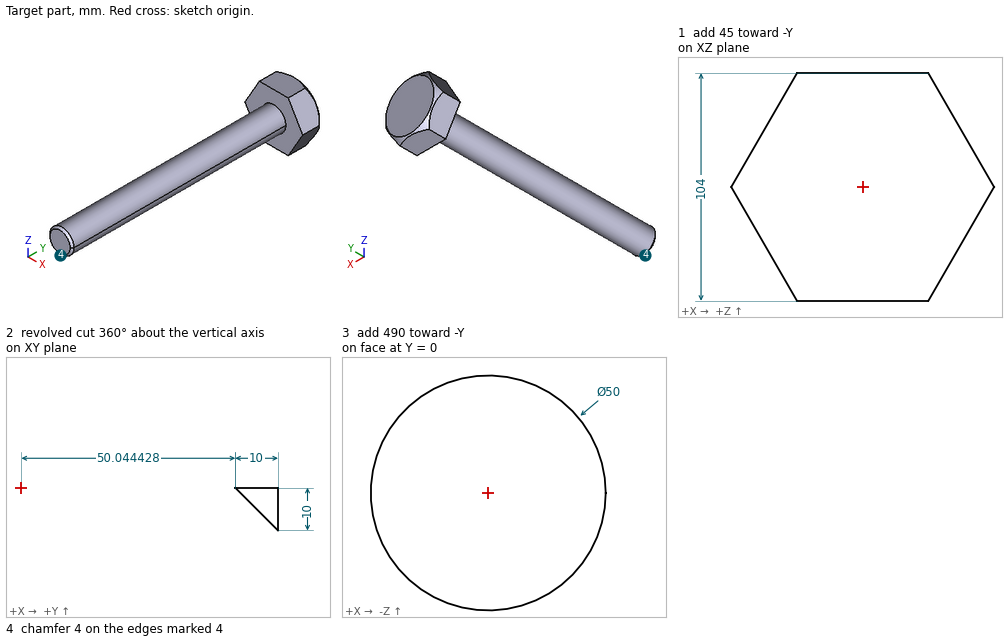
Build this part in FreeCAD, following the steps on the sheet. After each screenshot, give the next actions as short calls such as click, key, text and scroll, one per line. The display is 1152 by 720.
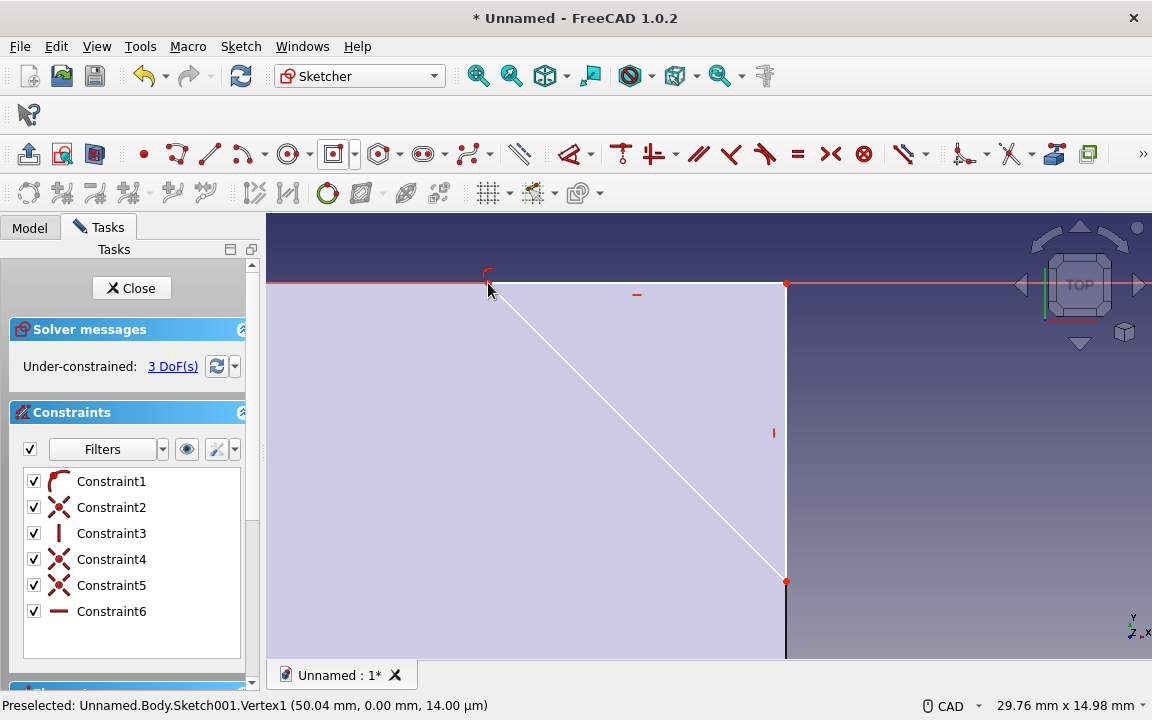
click(786, 492)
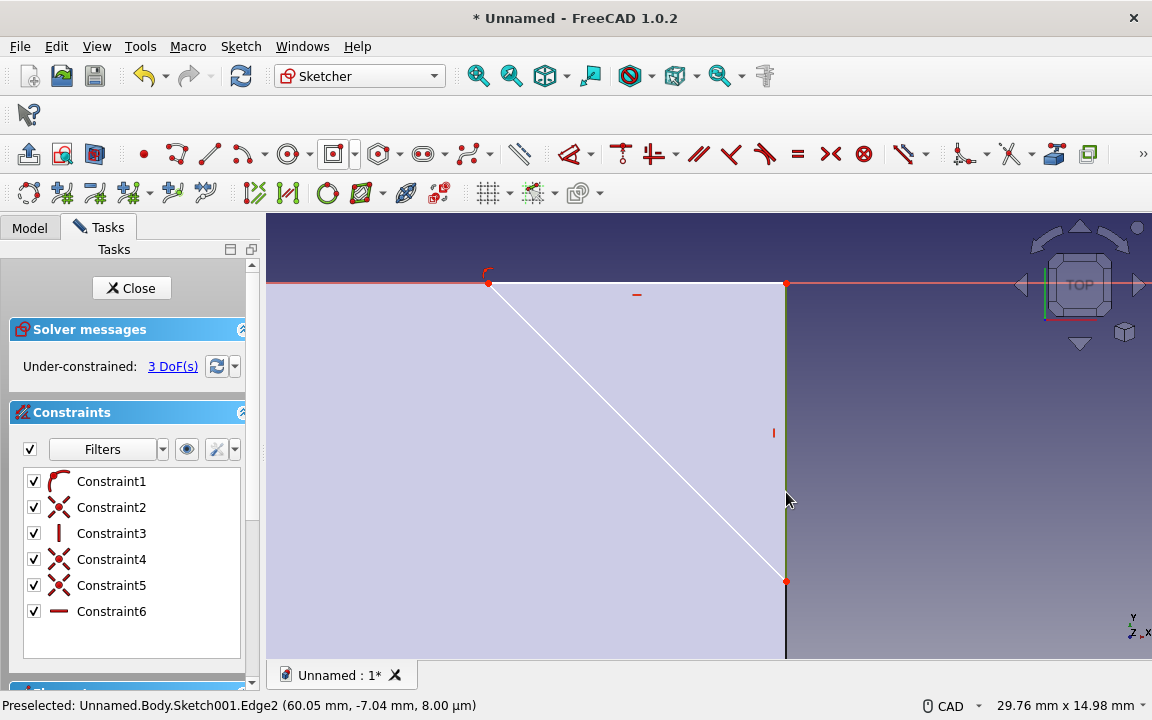
key(i)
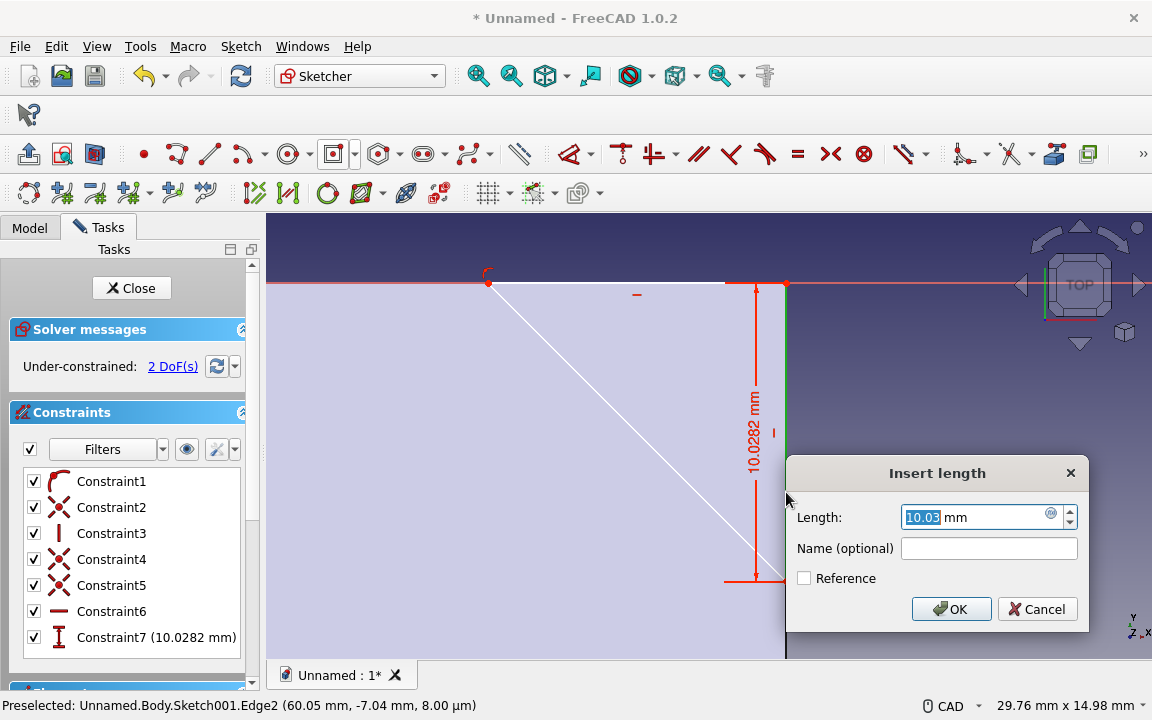
text(10)
key(Return)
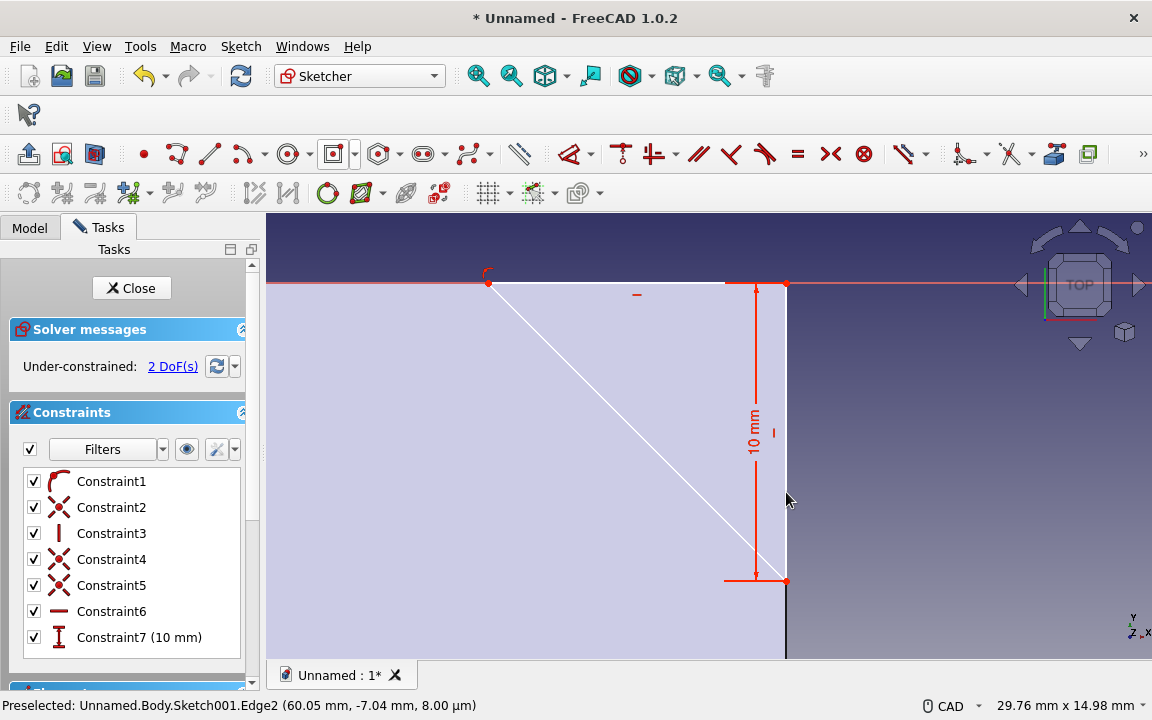
click(697, 283)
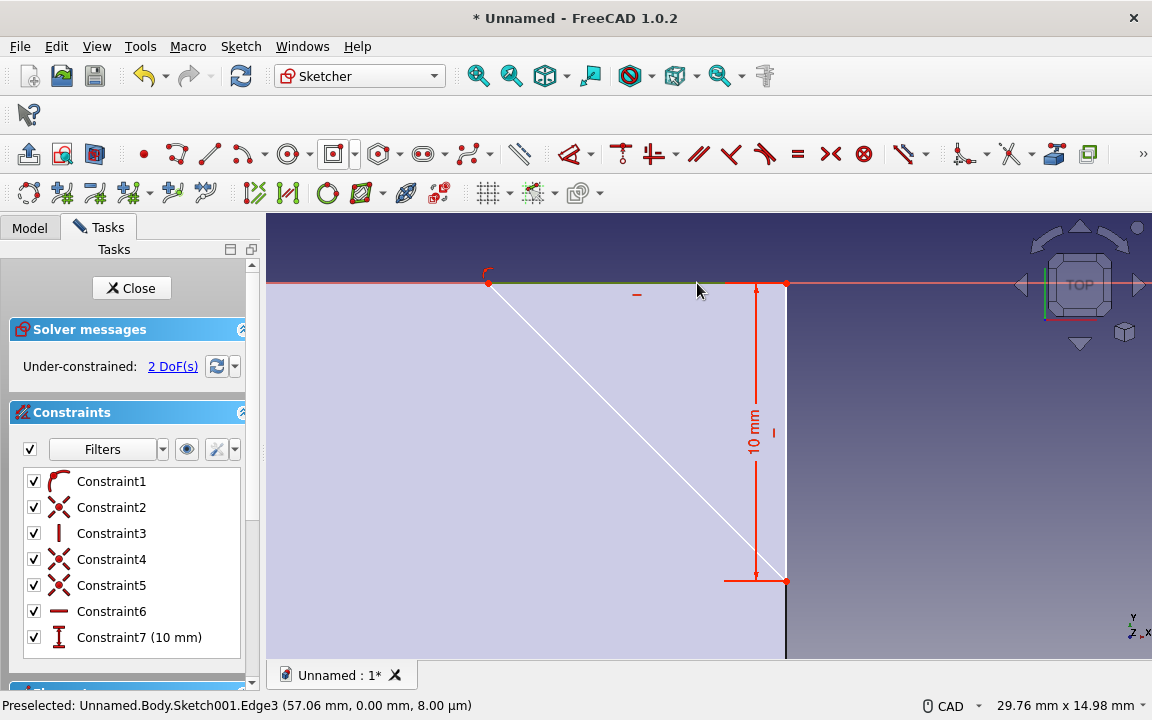
key(l)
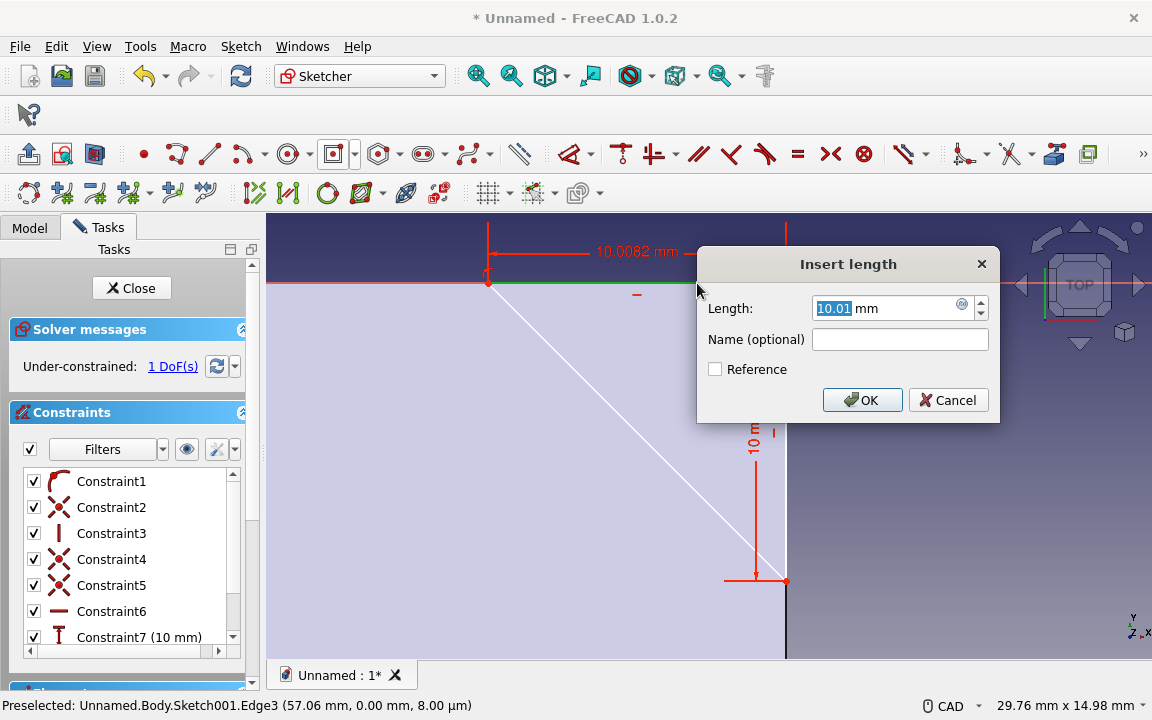
text(10)
key(Return)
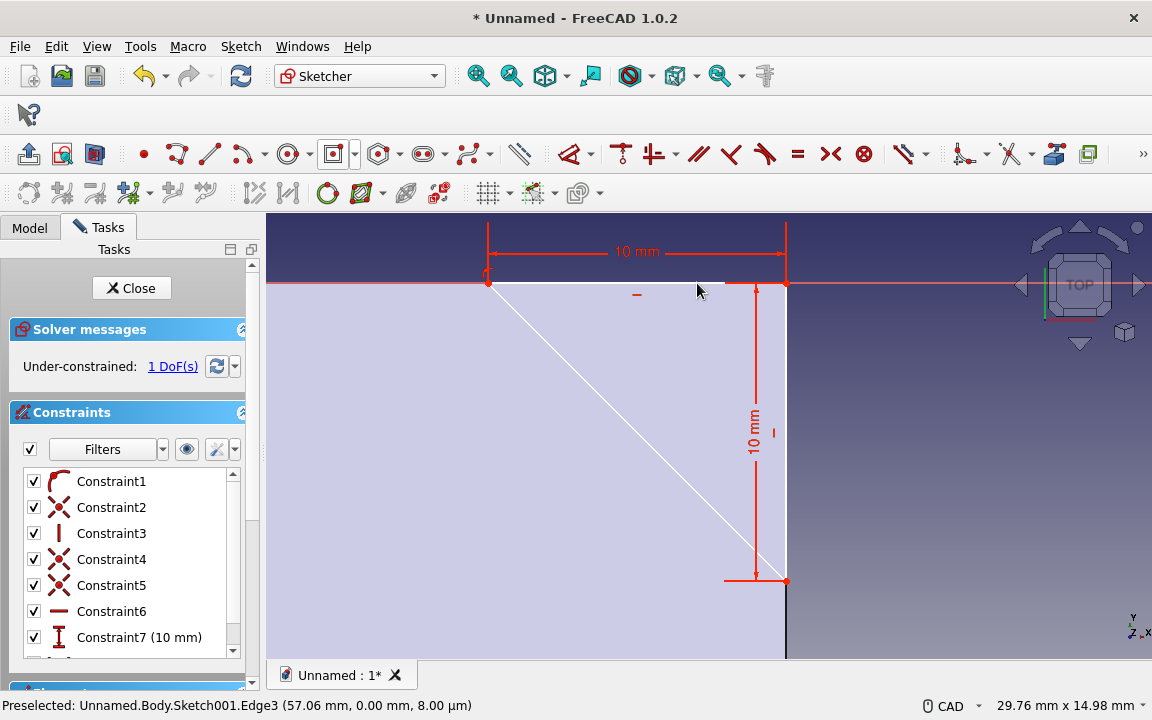
click(488, 283)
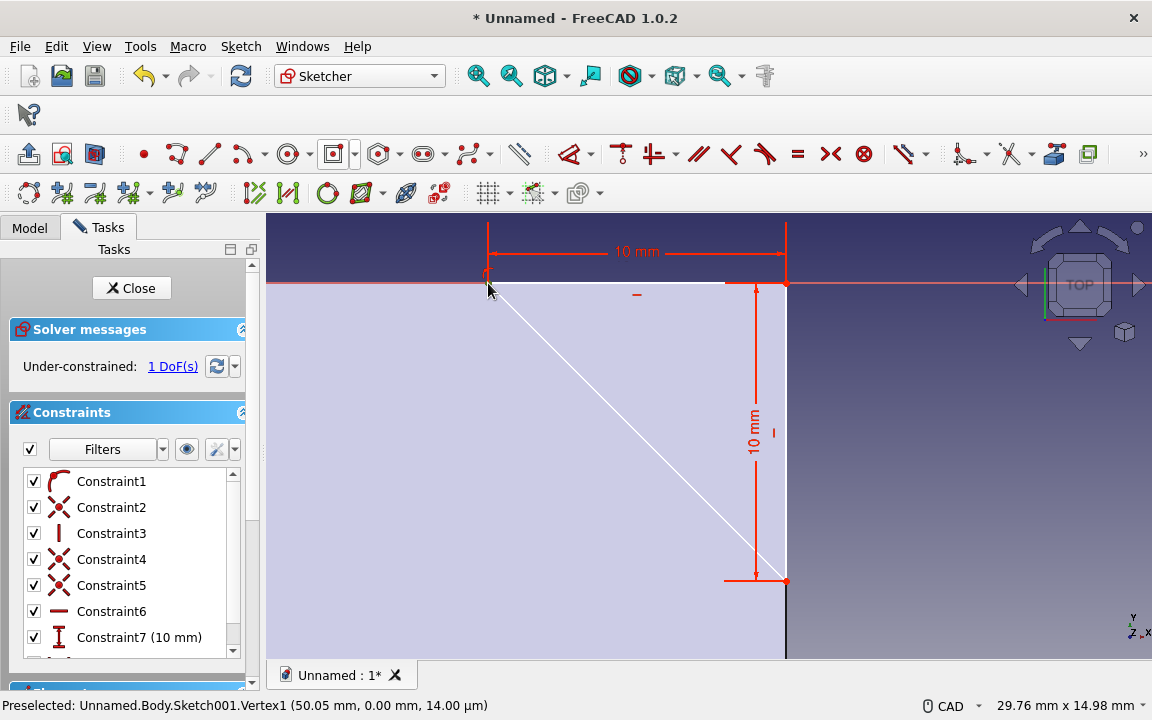
key(l)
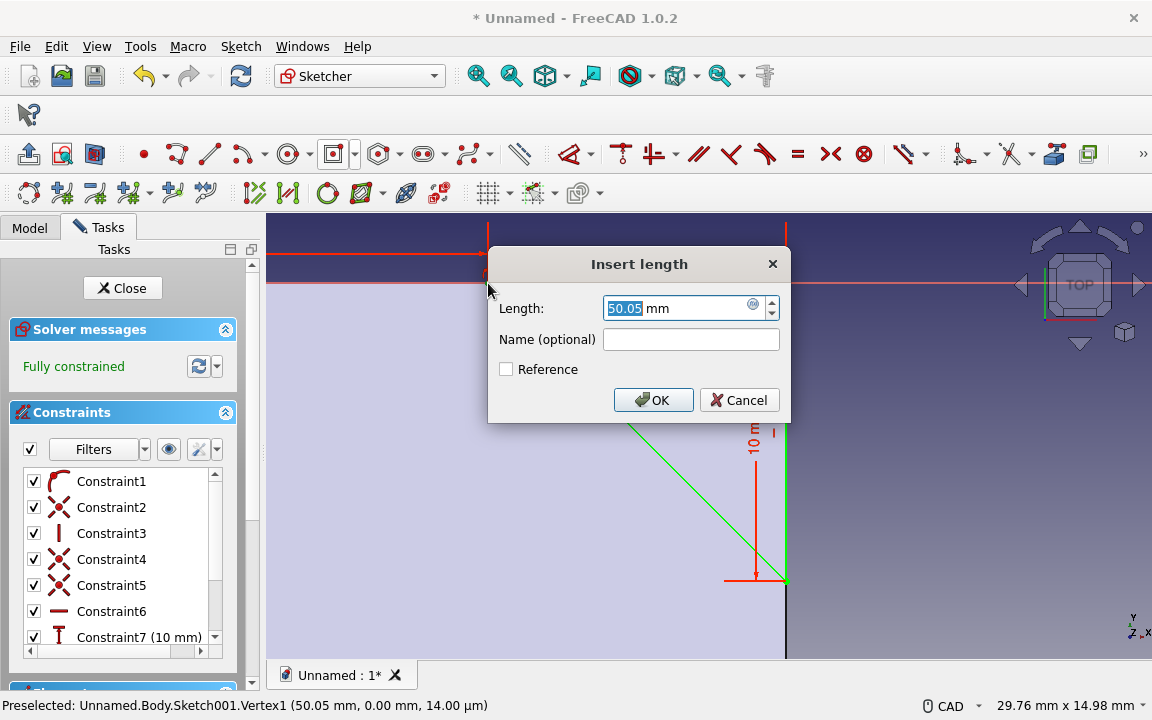
text(50.044428)
key(Return)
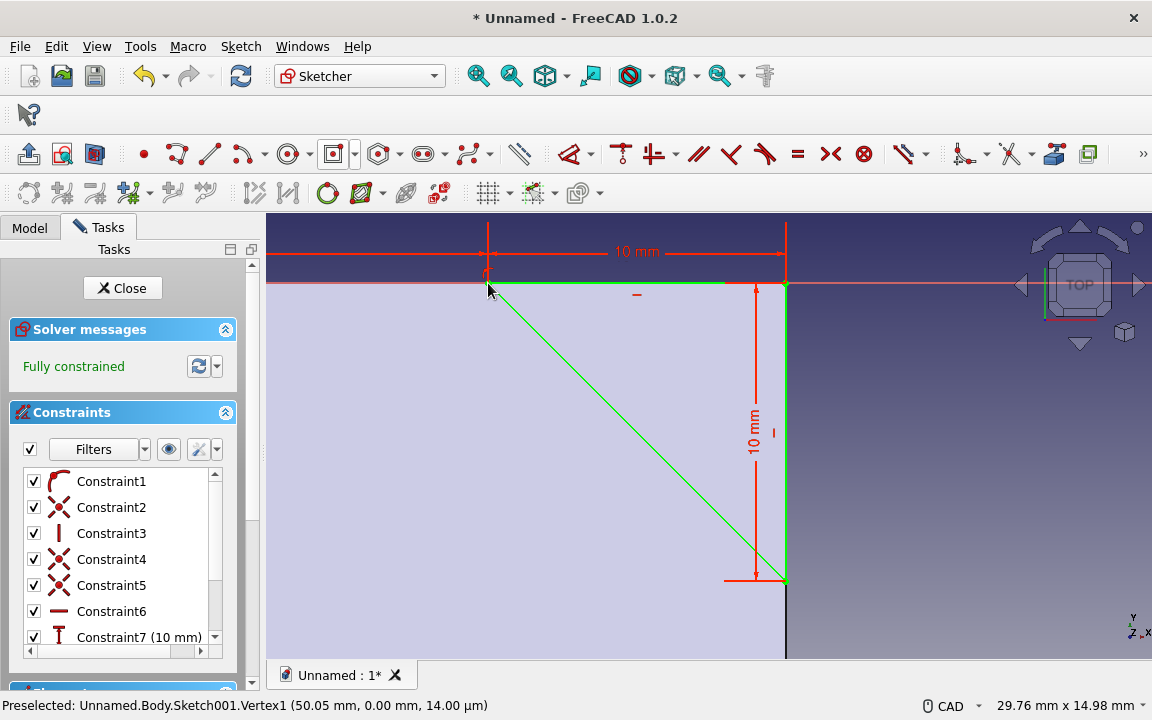
click(123, 288)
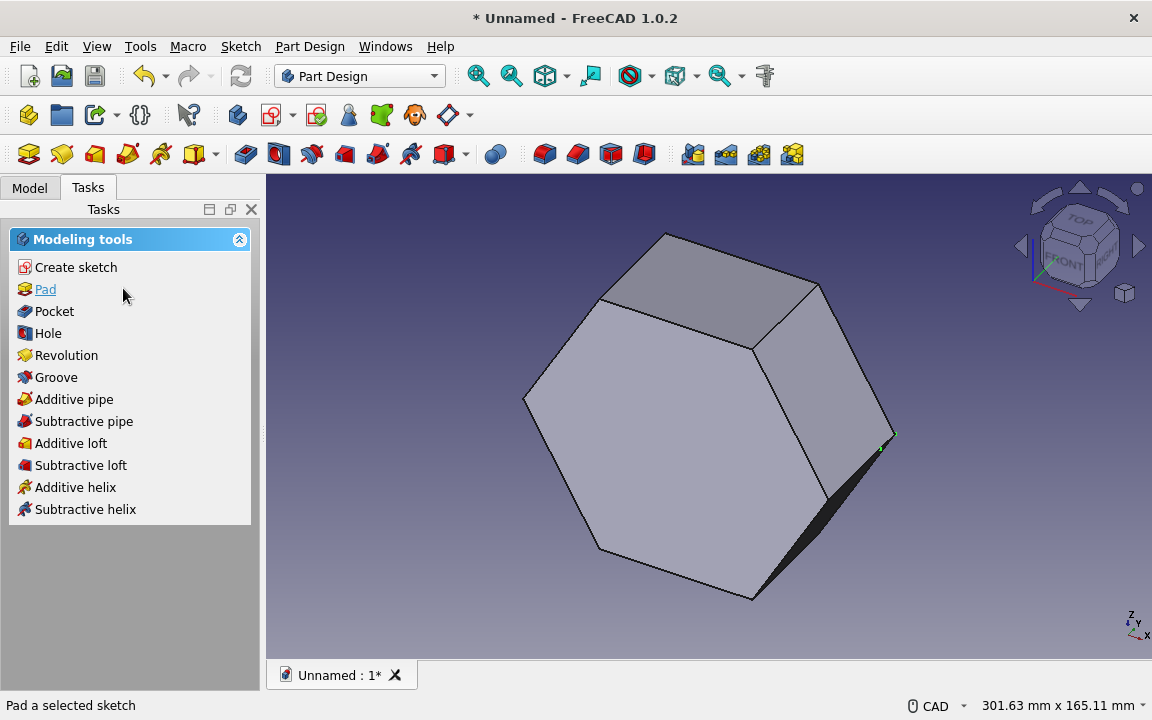
click(312, 154)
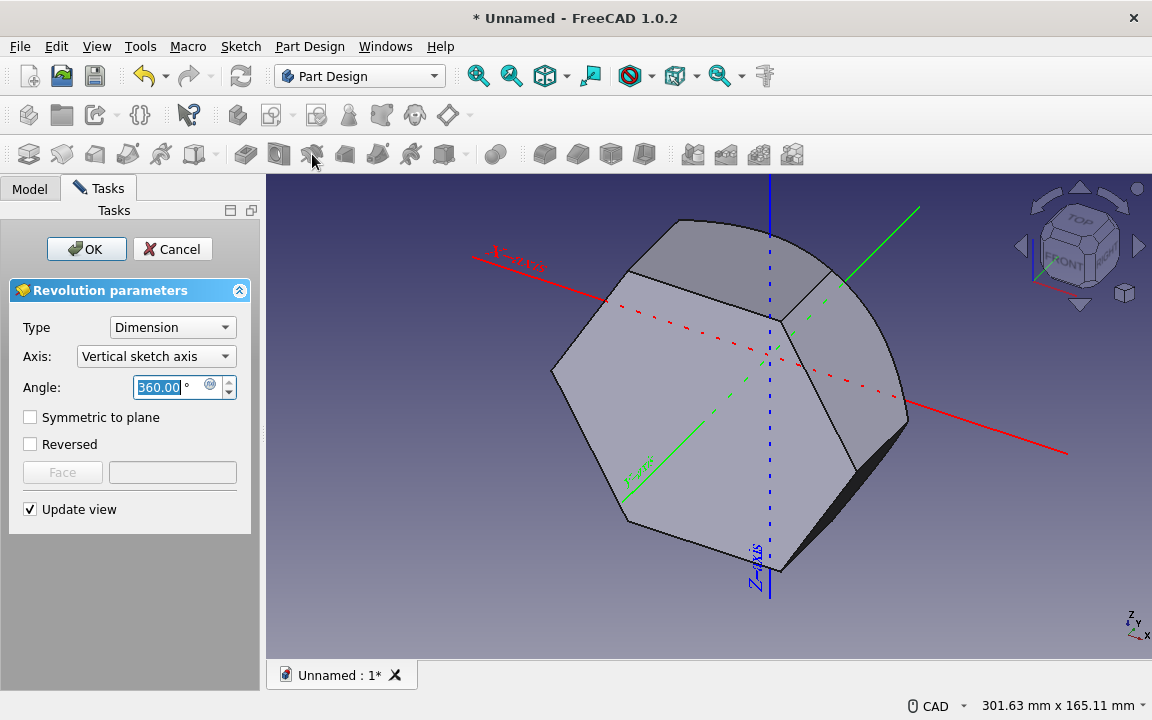
click(87, 249)